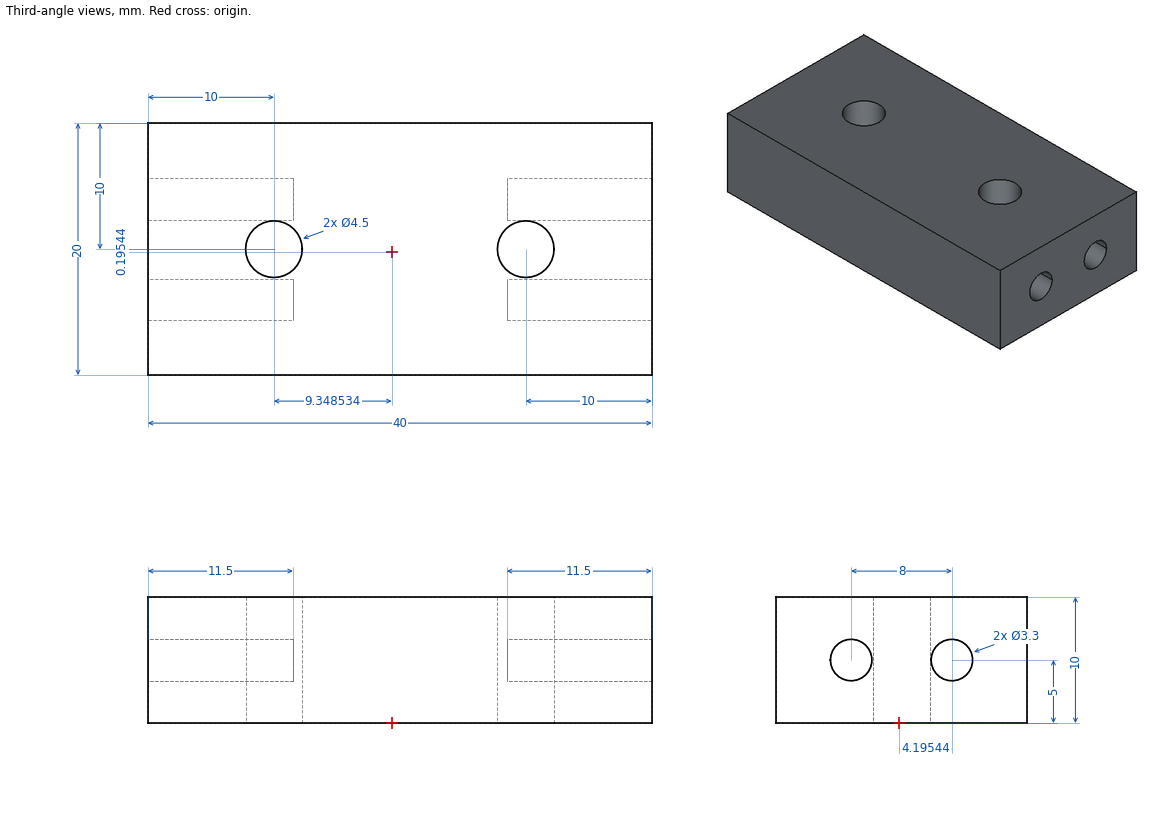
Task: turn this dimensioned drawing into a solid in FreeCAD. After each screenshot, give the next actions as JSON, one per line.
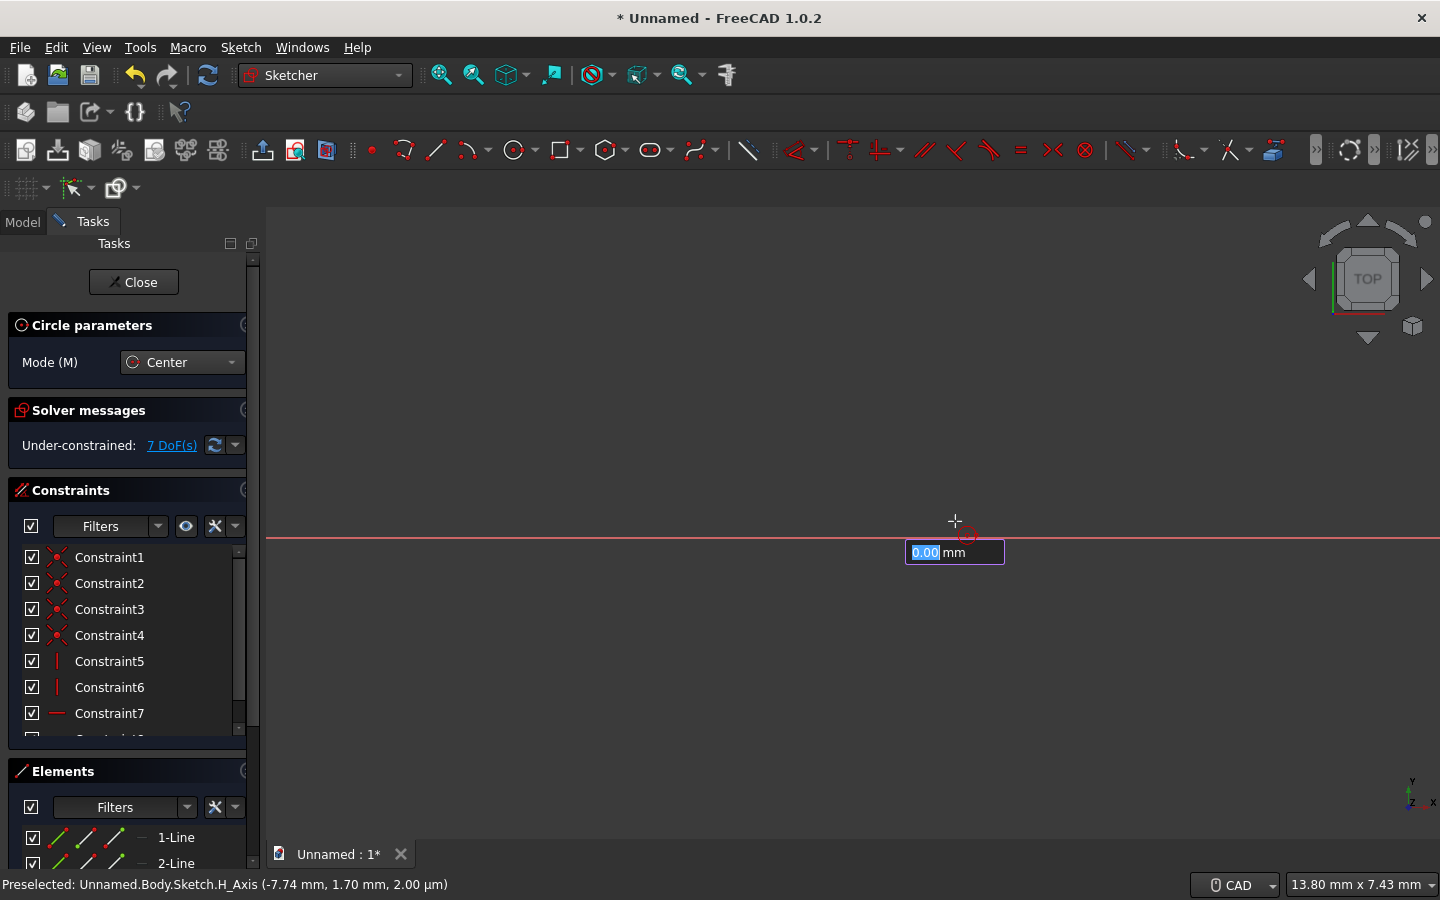
{"action": "scroll", "coordinate": [957, 523], "scroll_direction": "down", "scroll_amount": 8}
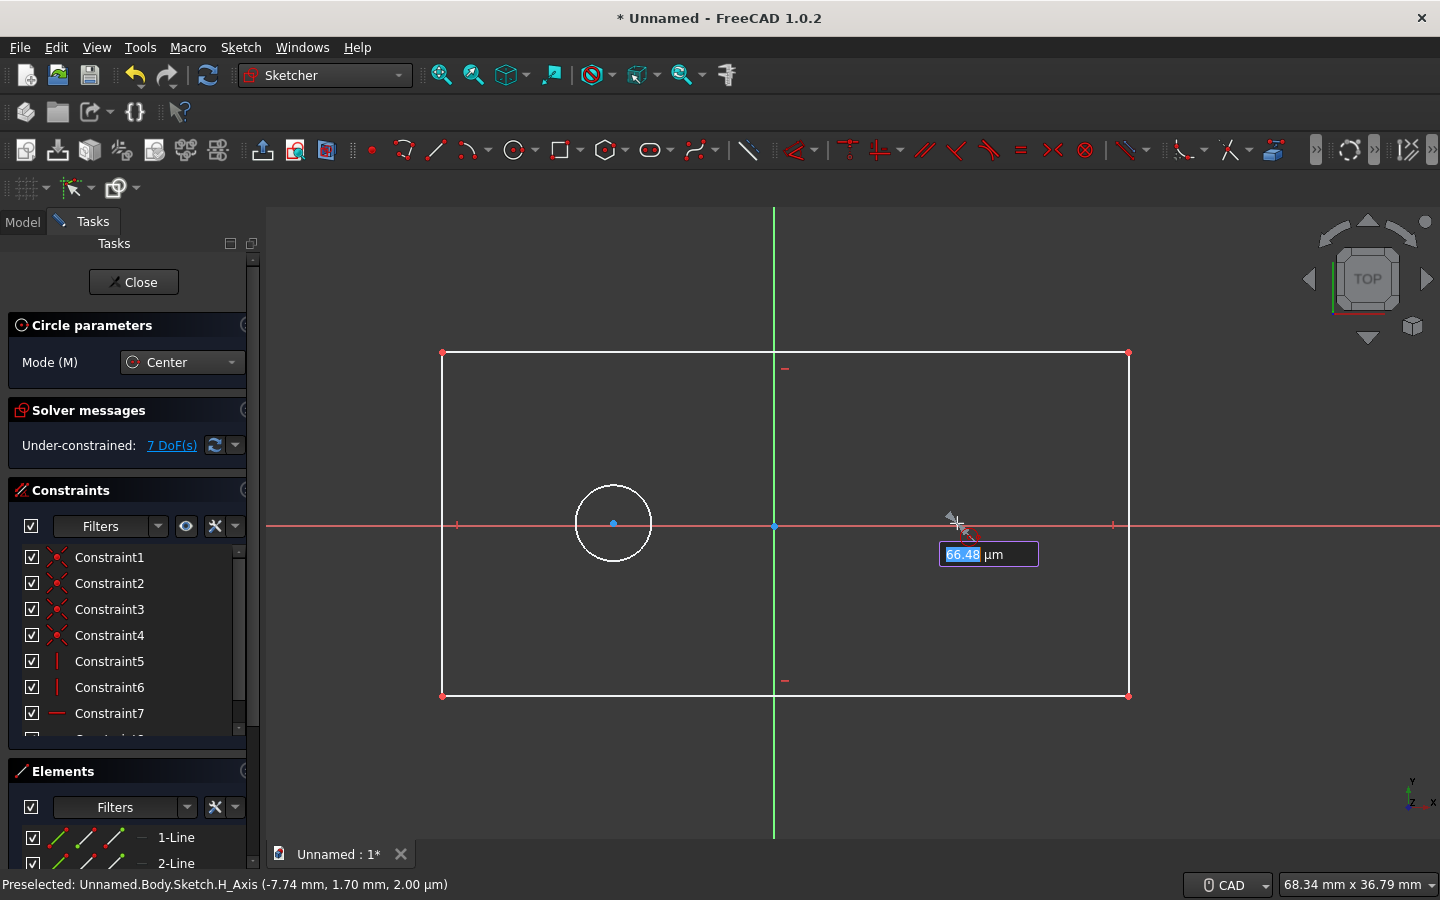
{"action": "left_click", "coordinate": [984, 496]}
{"action": "key", "text": "Escape"}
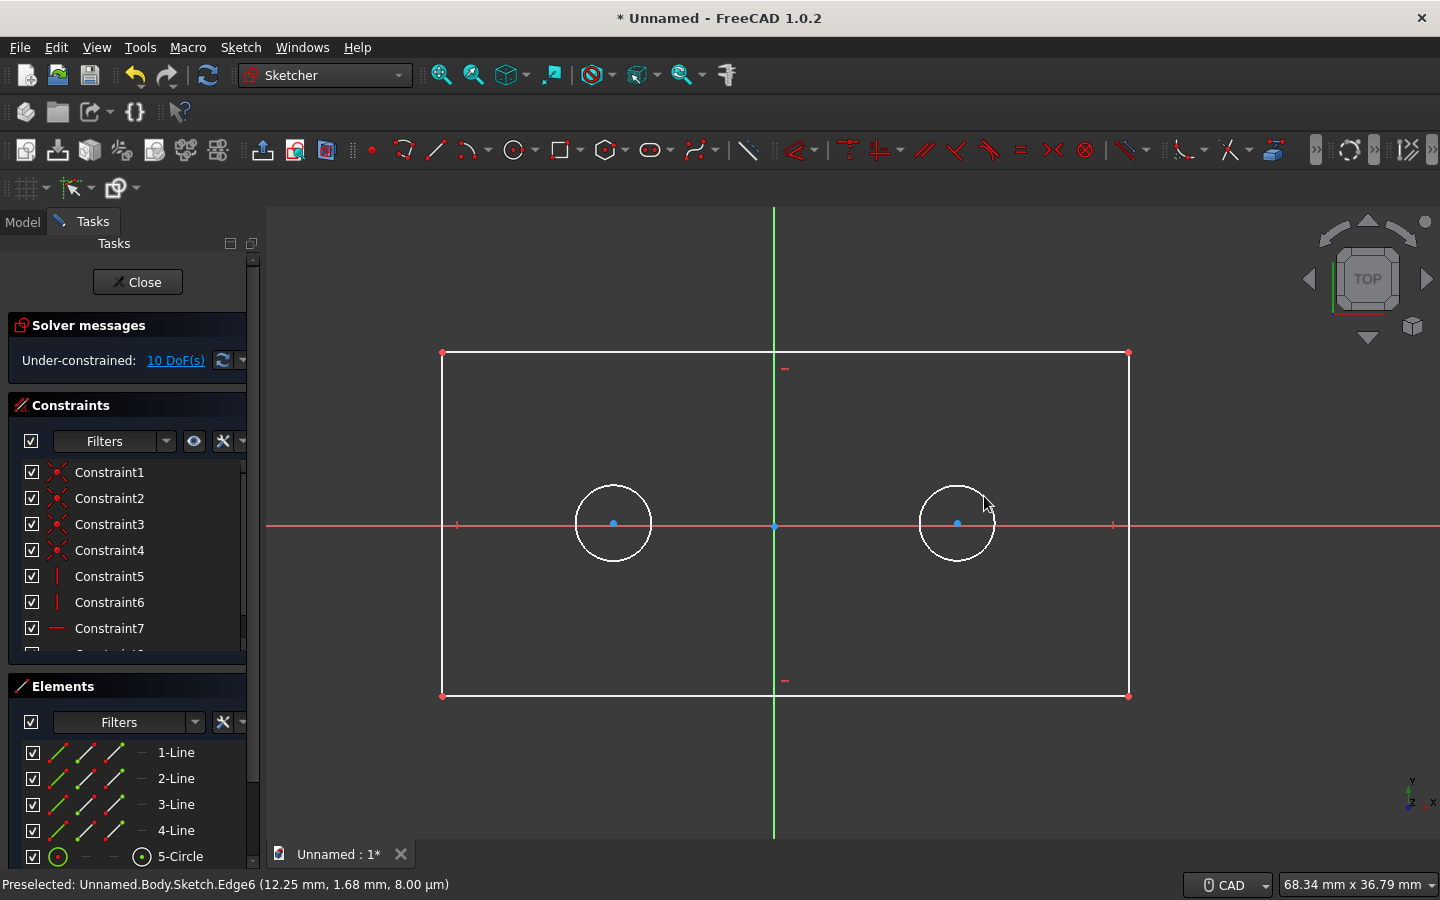
{"action": "left_click", "coordinate": [640, 496]}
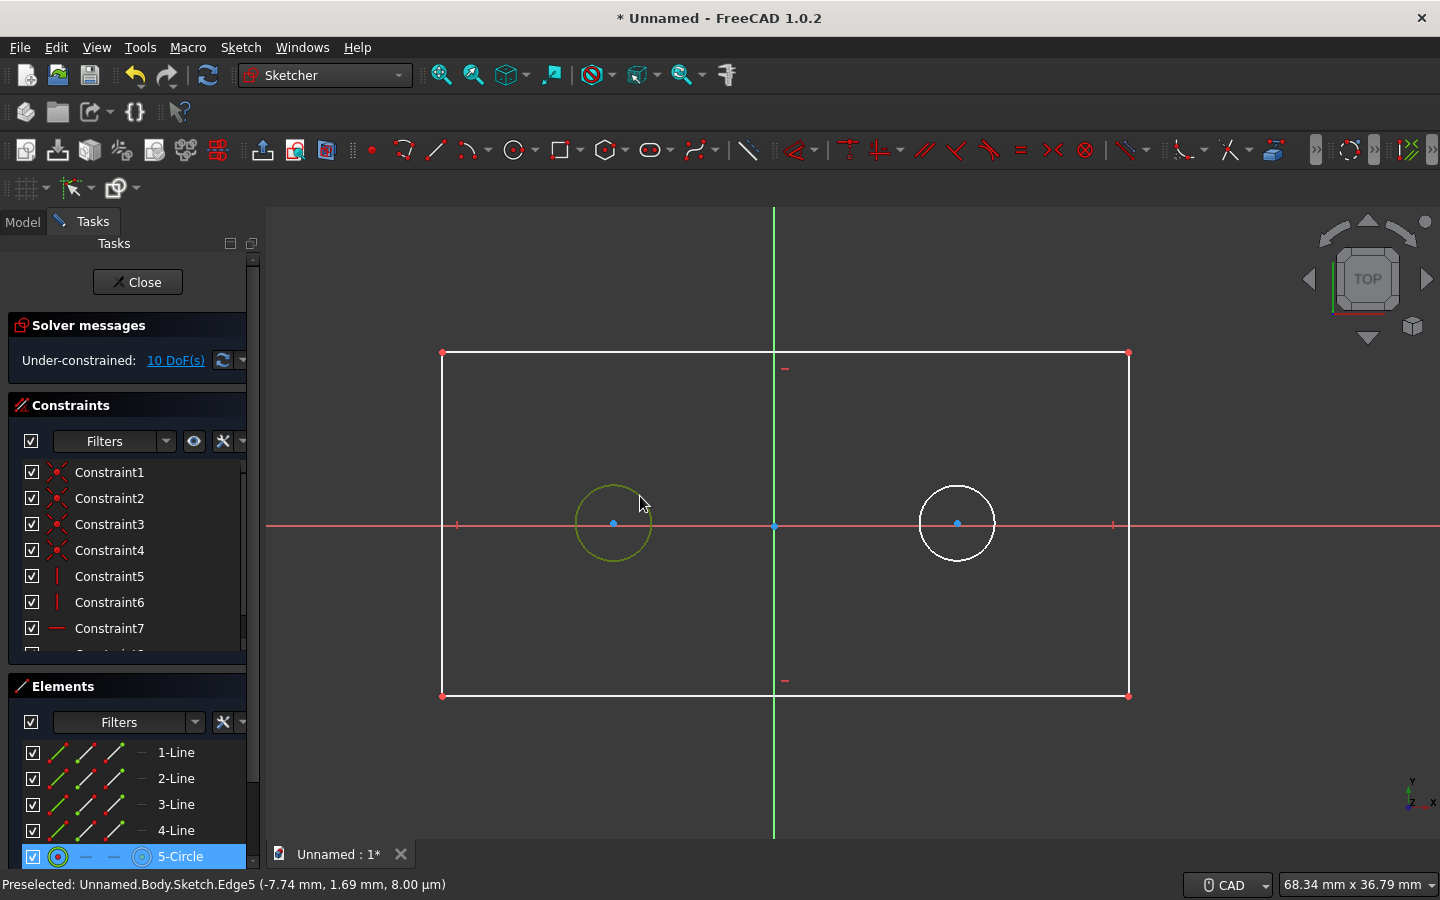
{"action": "left_click", "coordinate": [984, 497]}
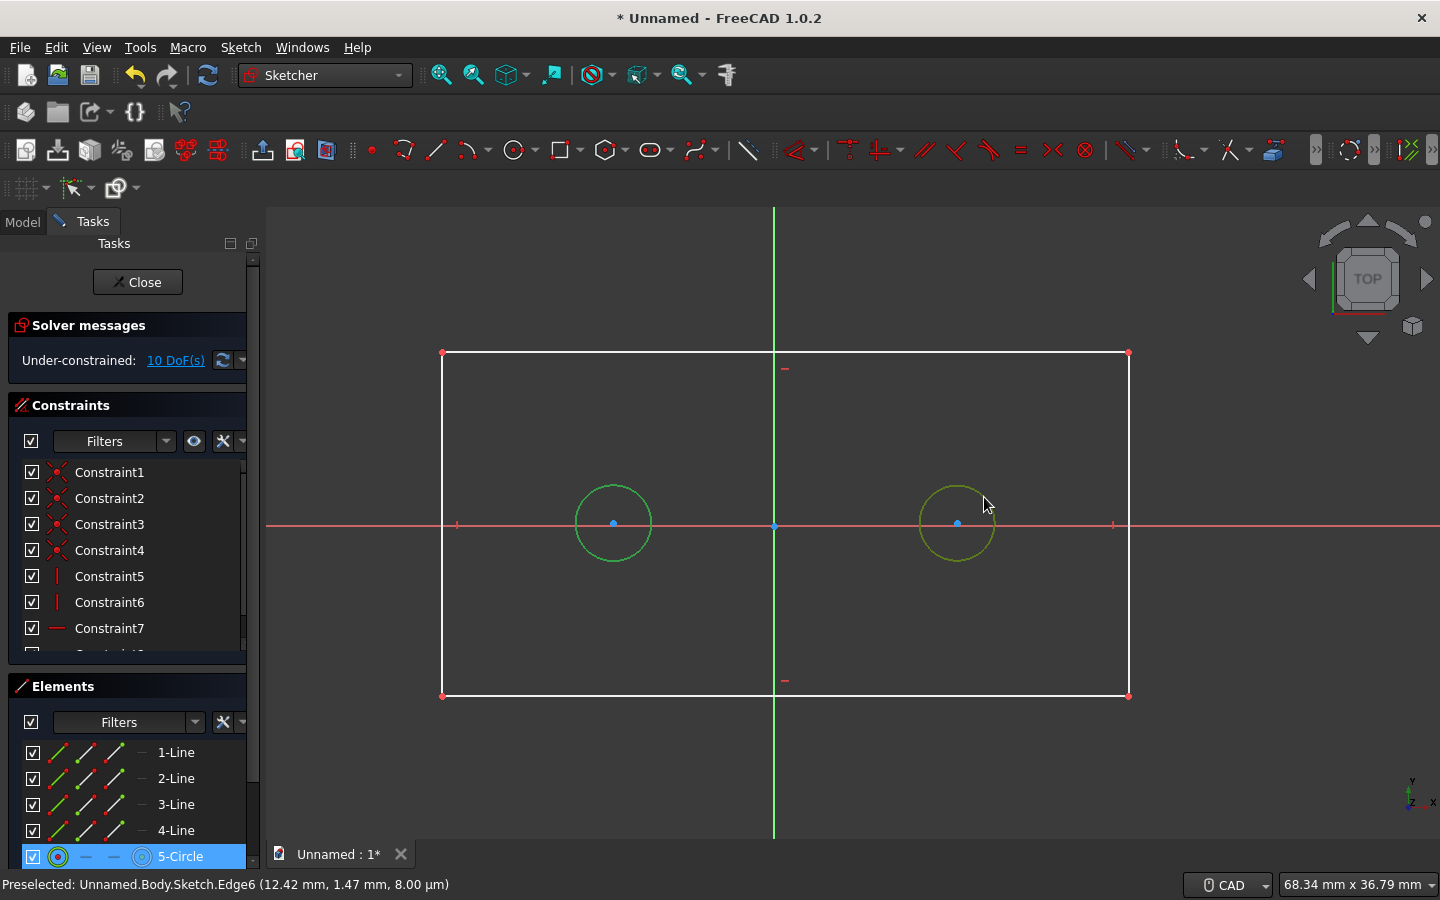
{"action": "key", "text": "e"}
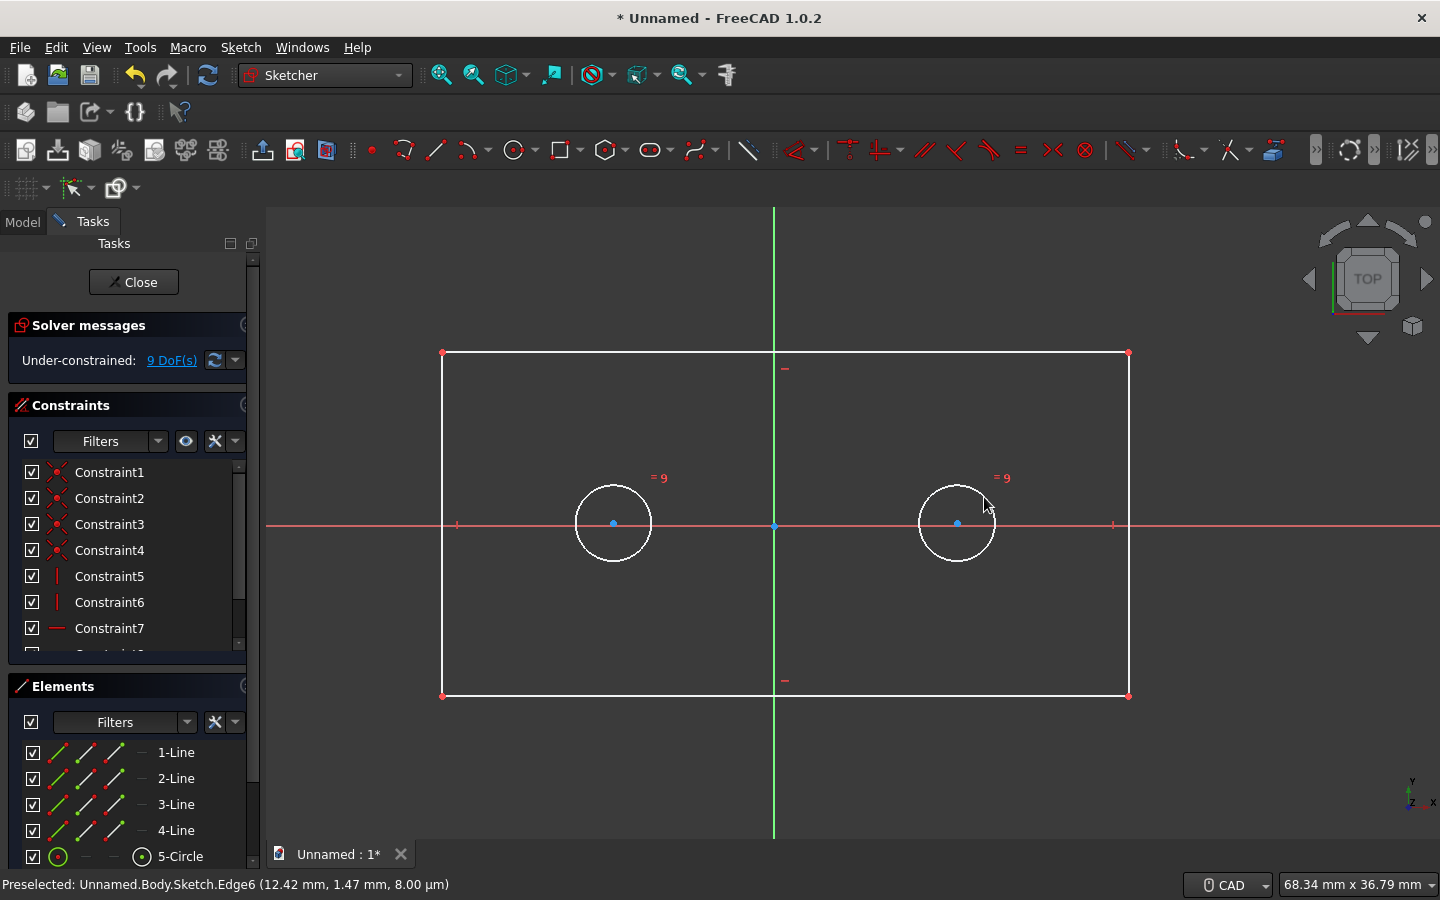
{"action": "left_click", "coordinate": [613, 523]}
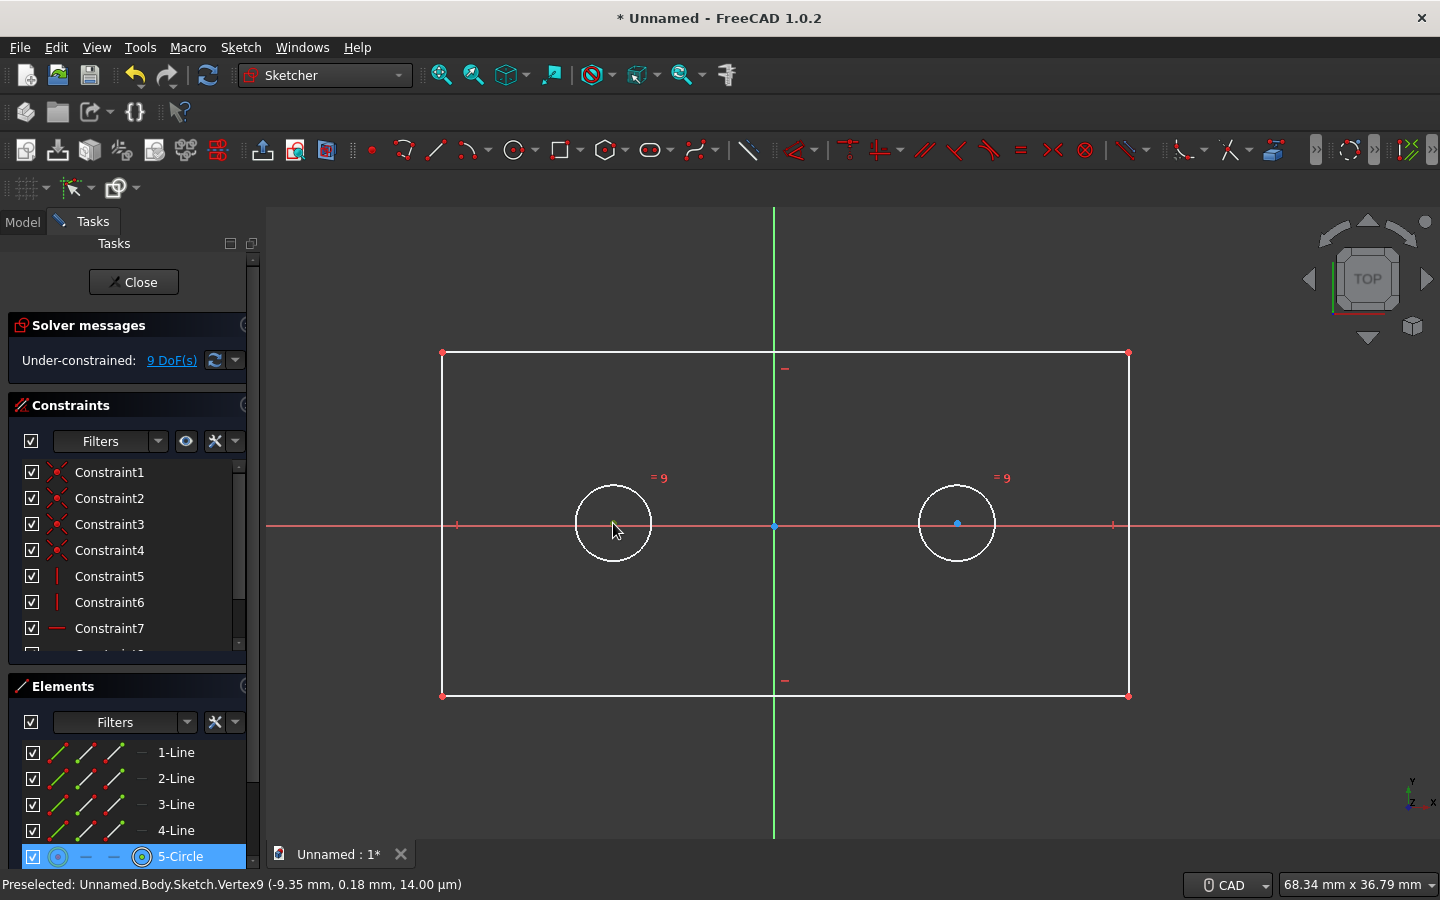
{"action": "left_click", "coordinate": [957, 523]}